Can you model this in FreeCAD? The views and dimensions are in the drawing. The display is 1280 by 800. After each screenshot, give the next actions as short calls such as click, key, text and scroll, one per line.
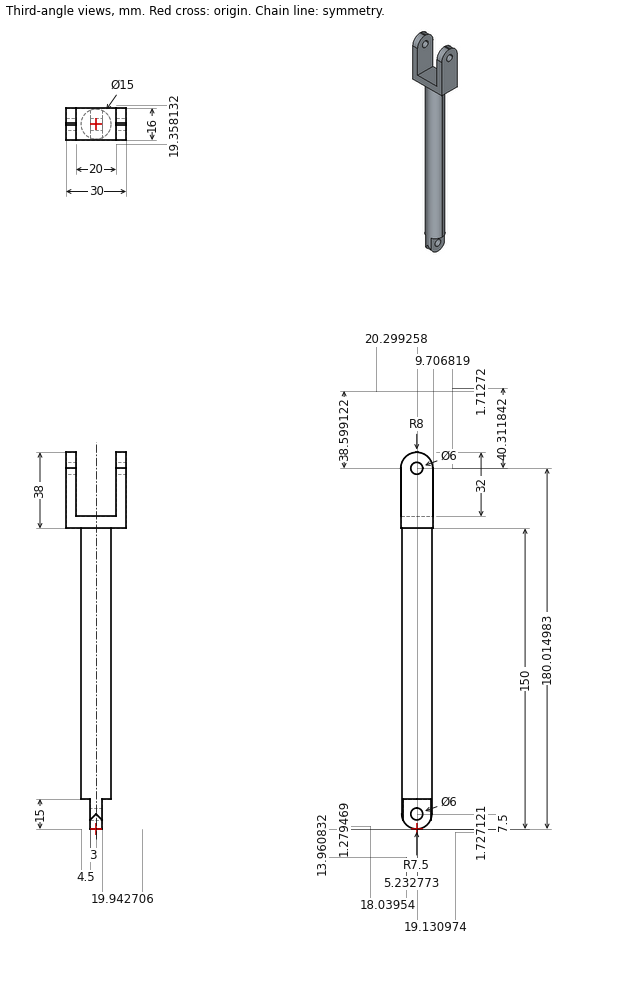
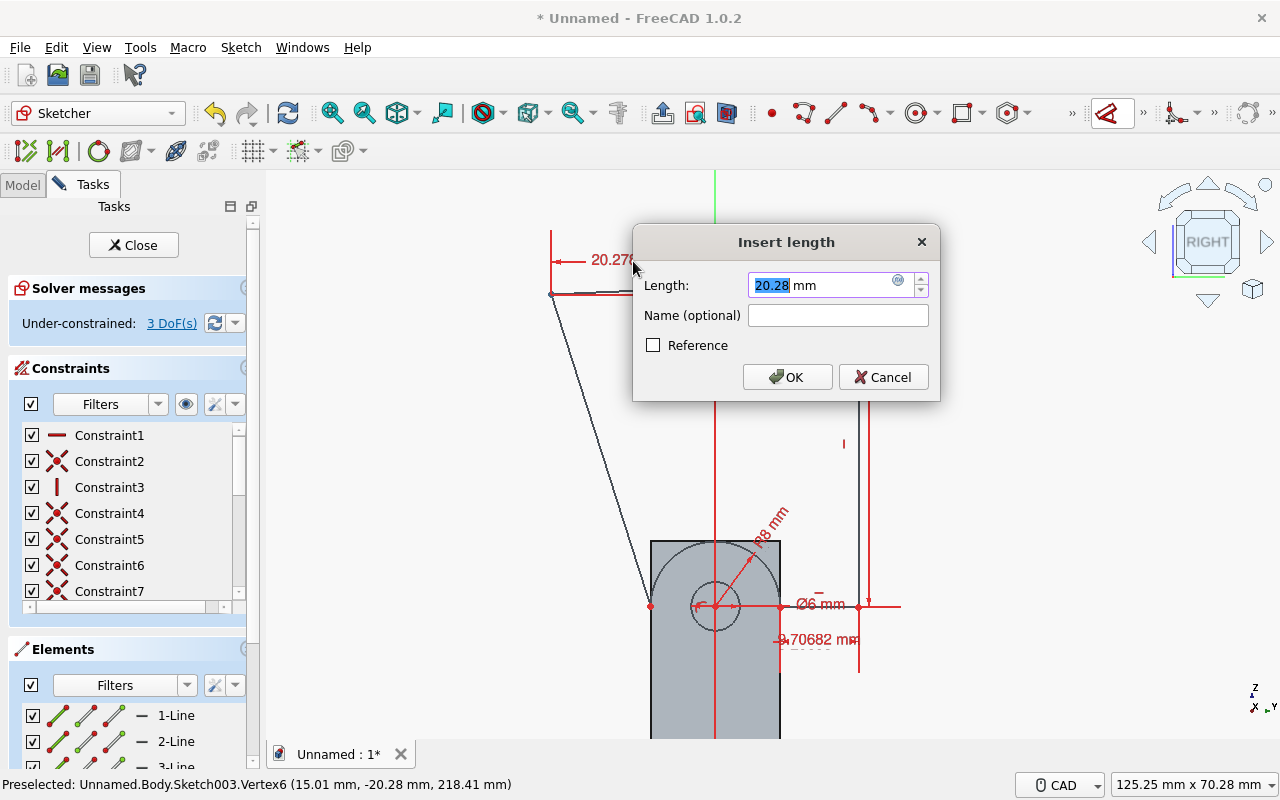
text(20.299258)
key(Return)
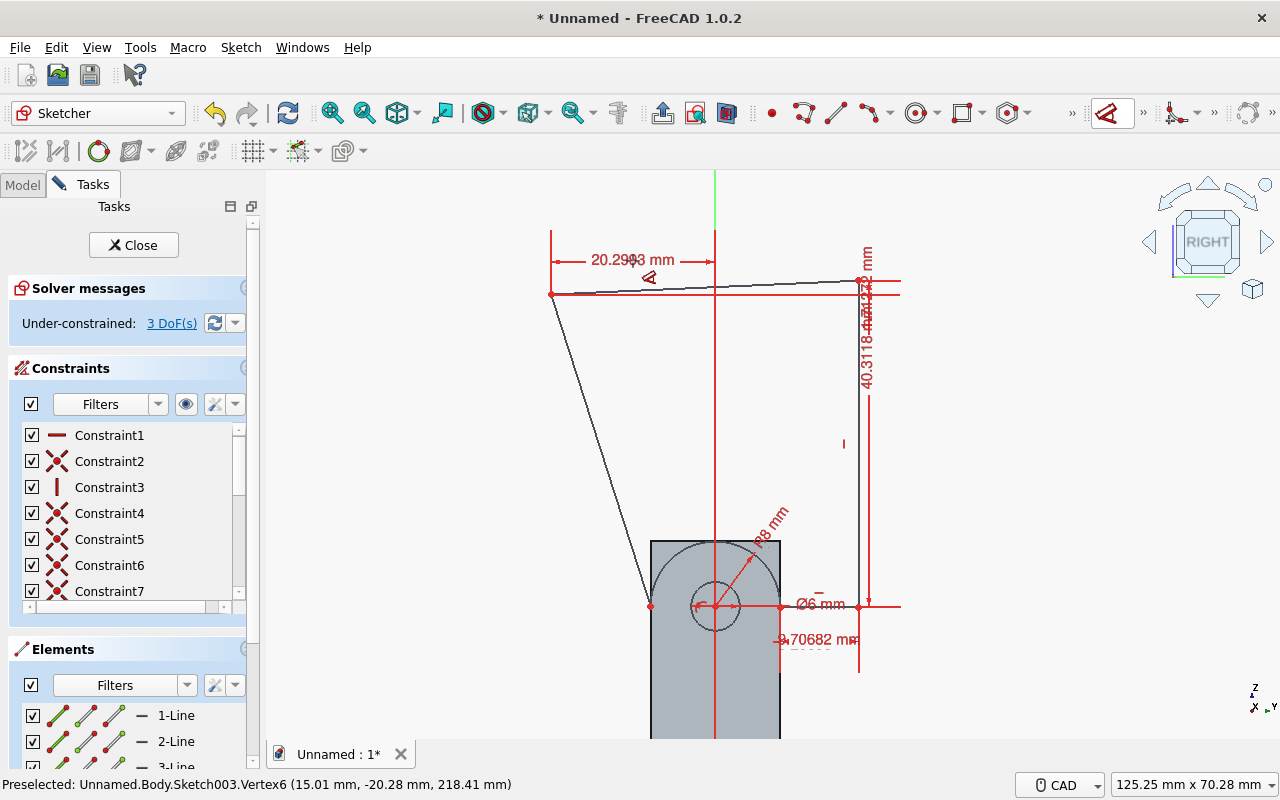
click(581, 388)
click(517, 450)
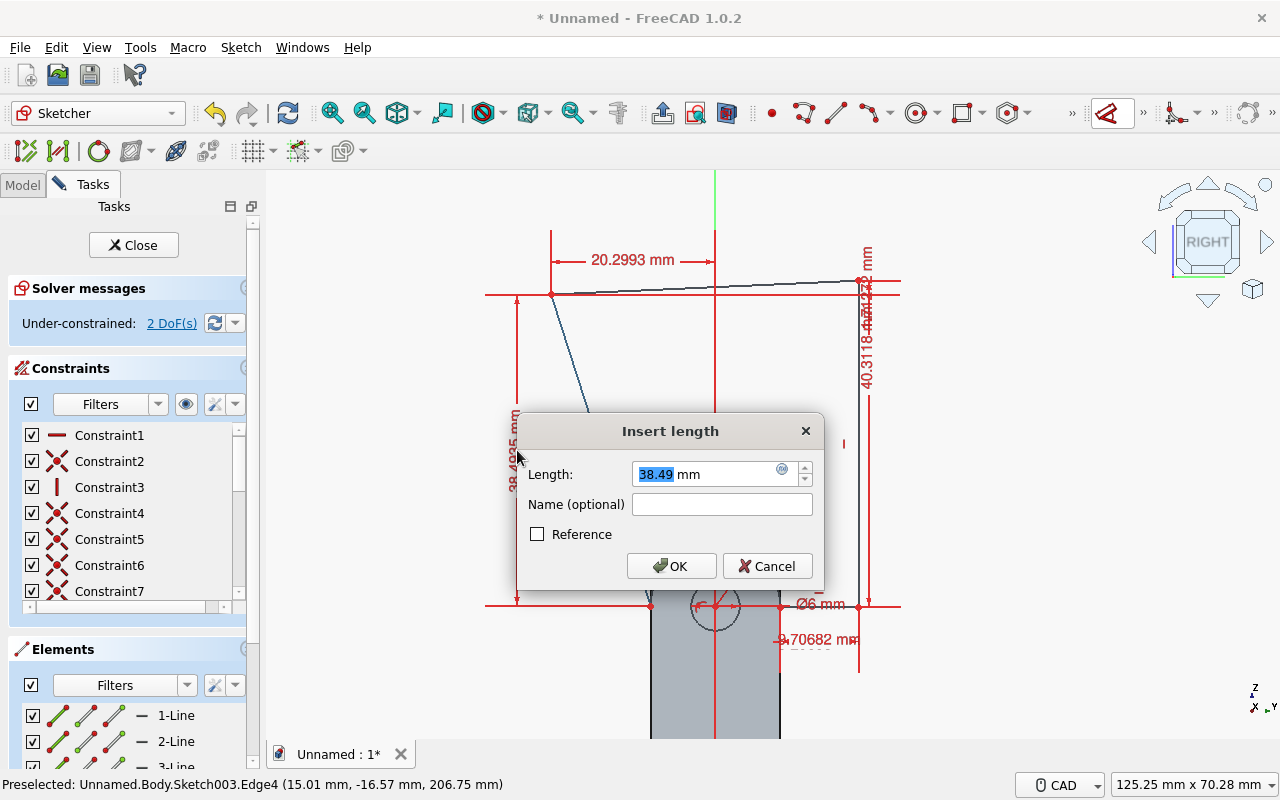
text(38.599122)
key(Return)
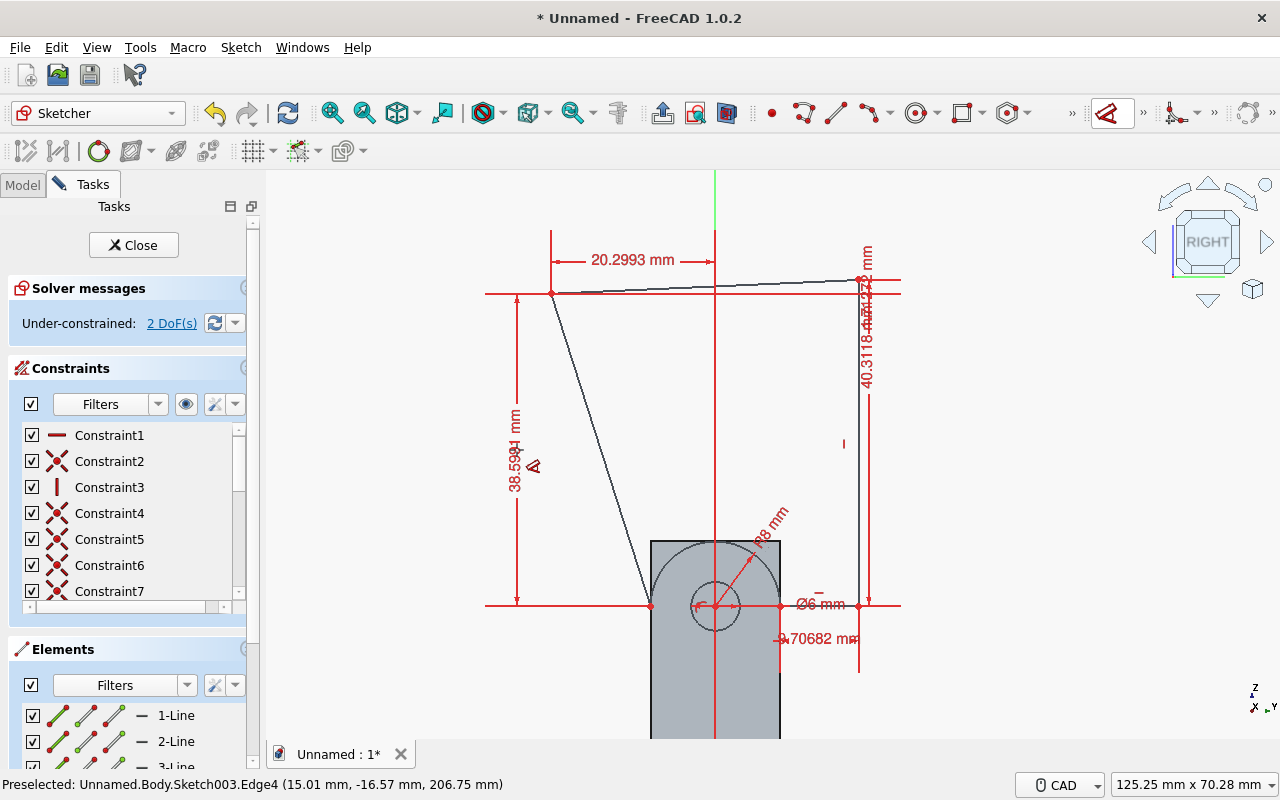
click(715, 606)
click(749, 659)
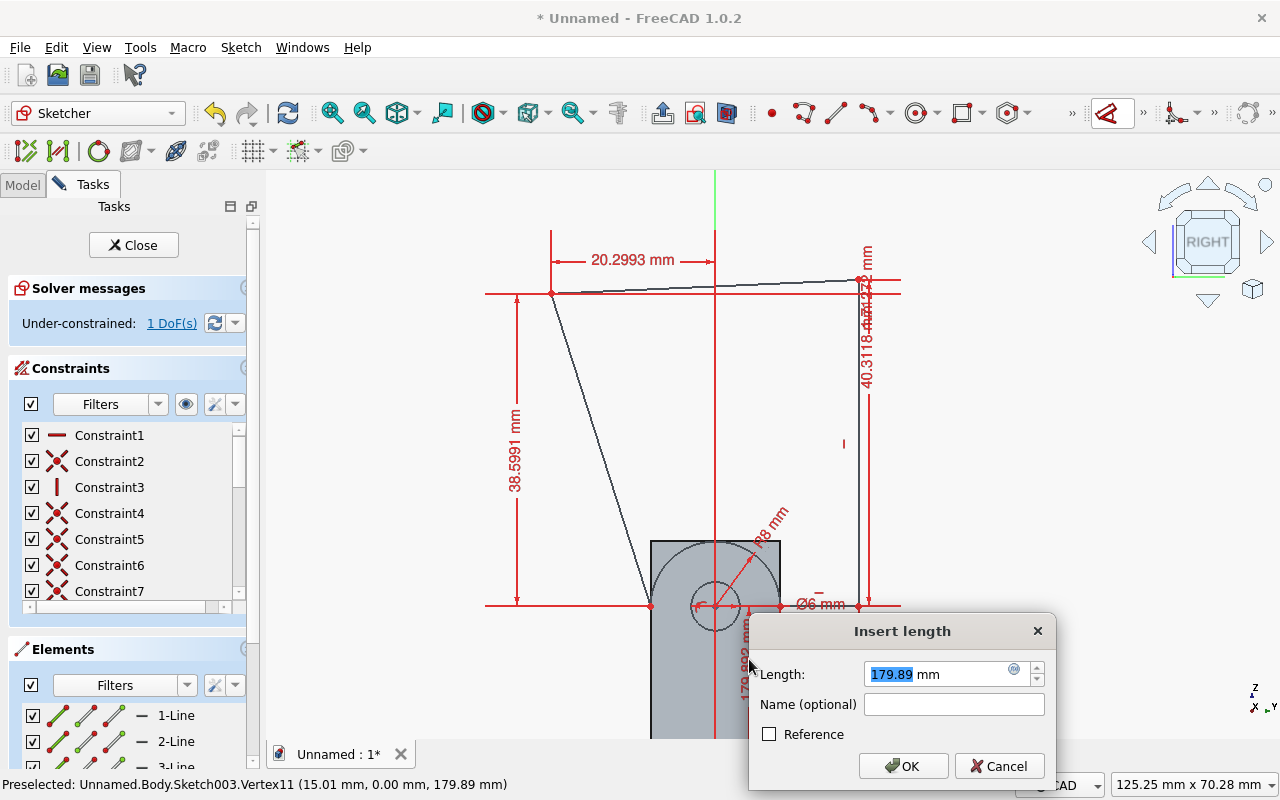
text(180.014983)
key(Return)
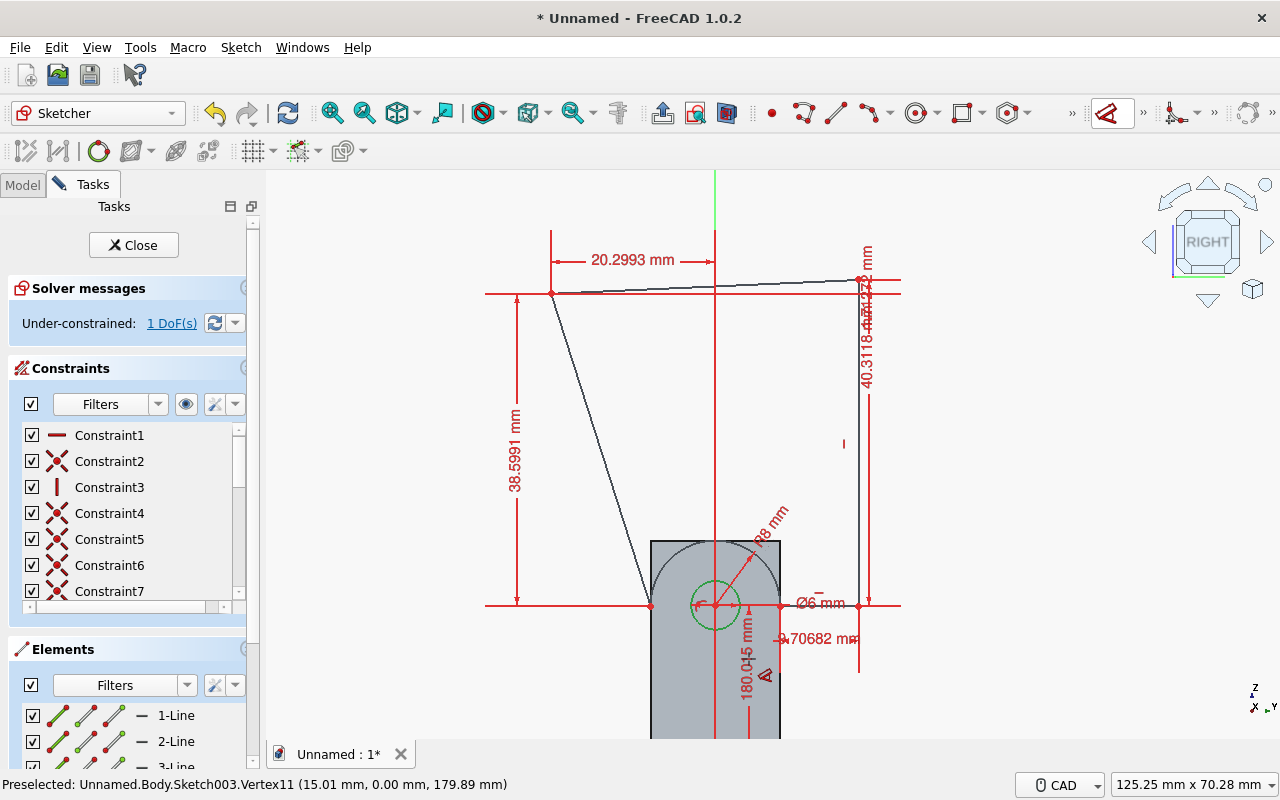
click(780, 606)
click(814, 683)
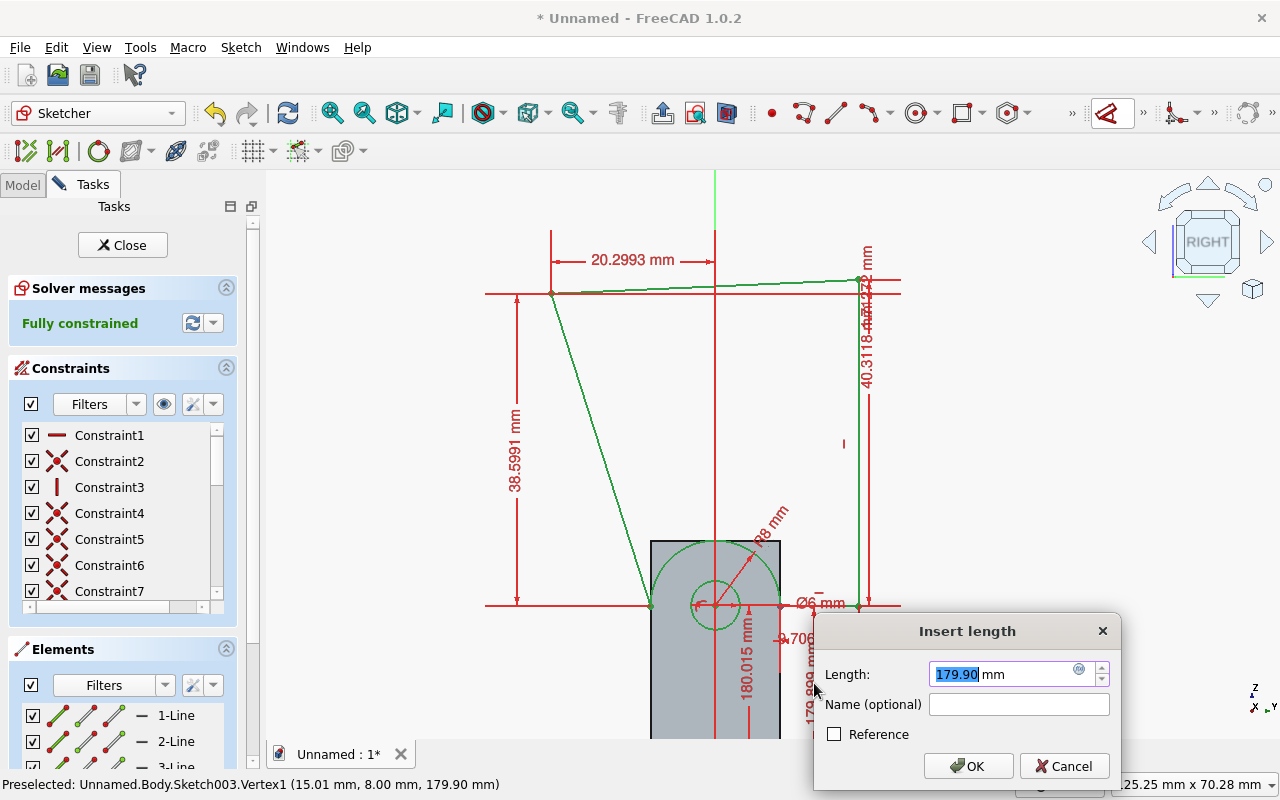
text(180.014983)
key(Return)
key(Escape)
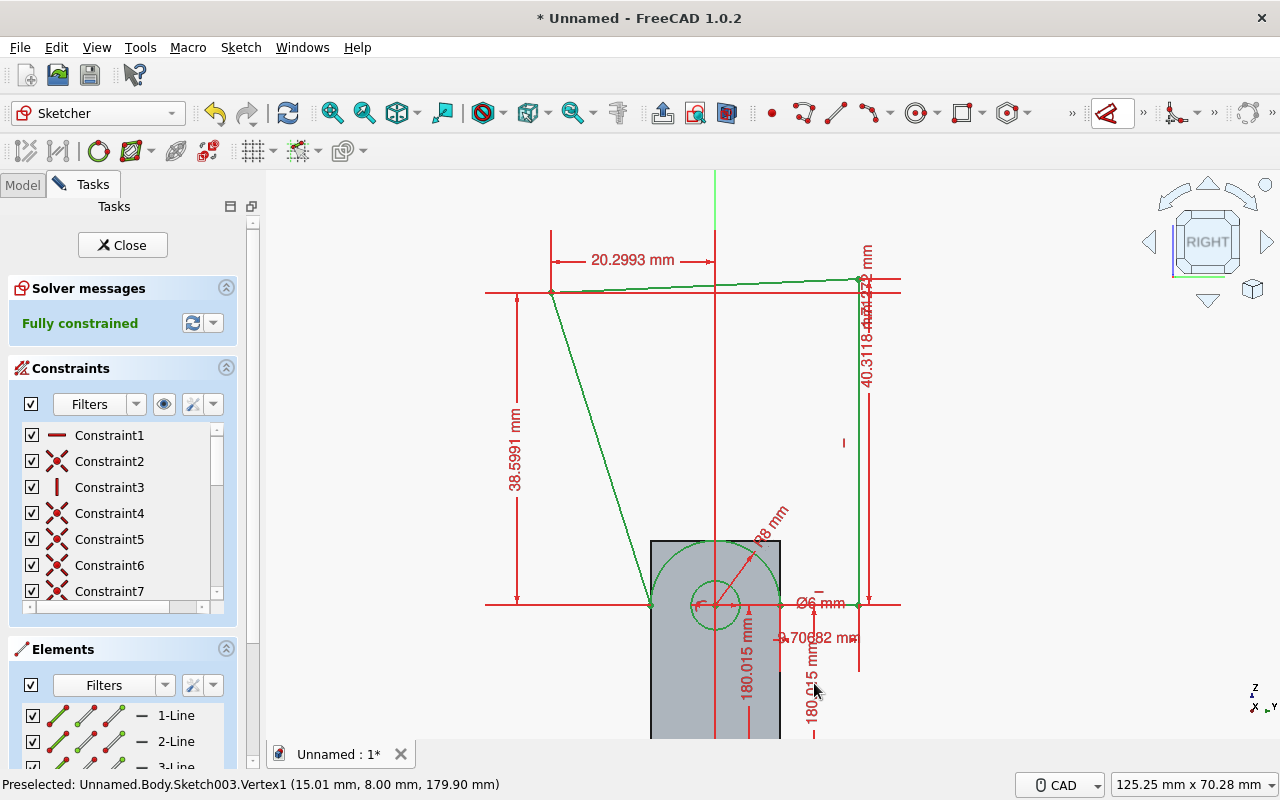
click(123, 245)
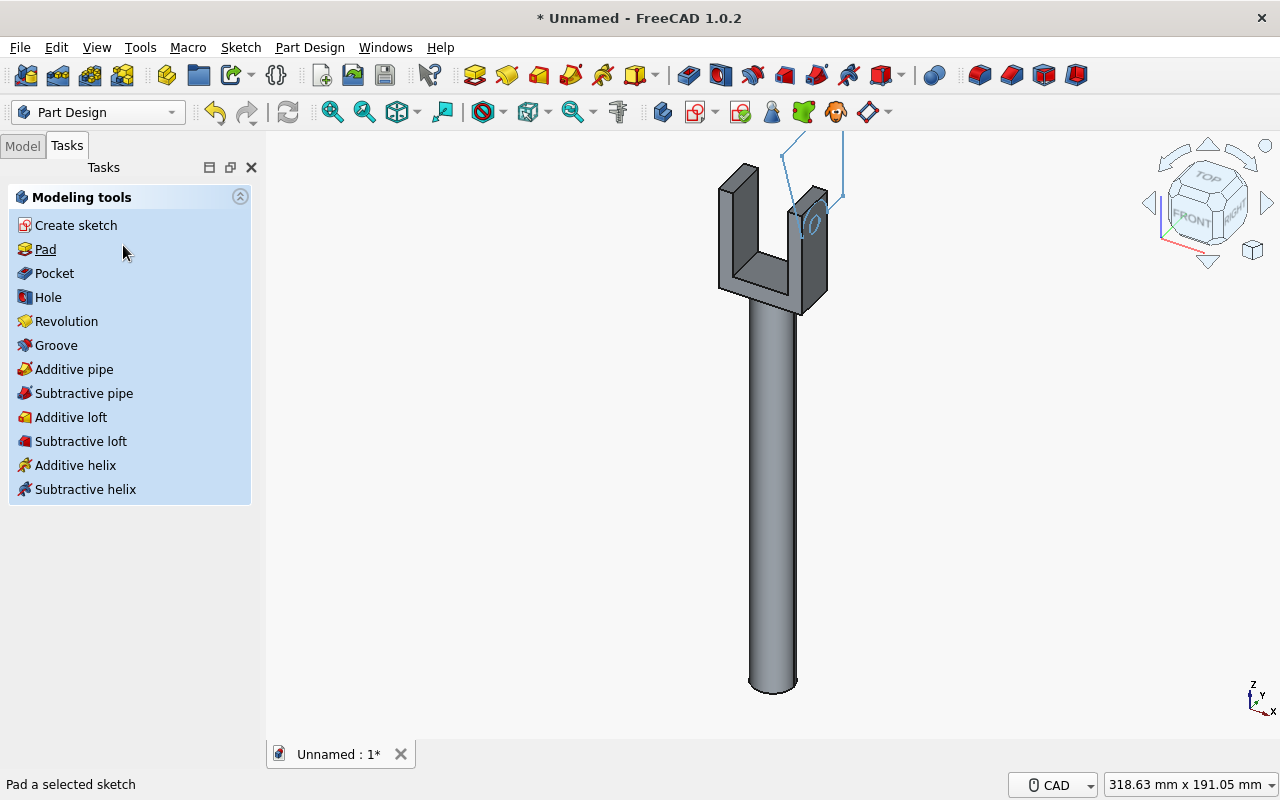
click(690, 76)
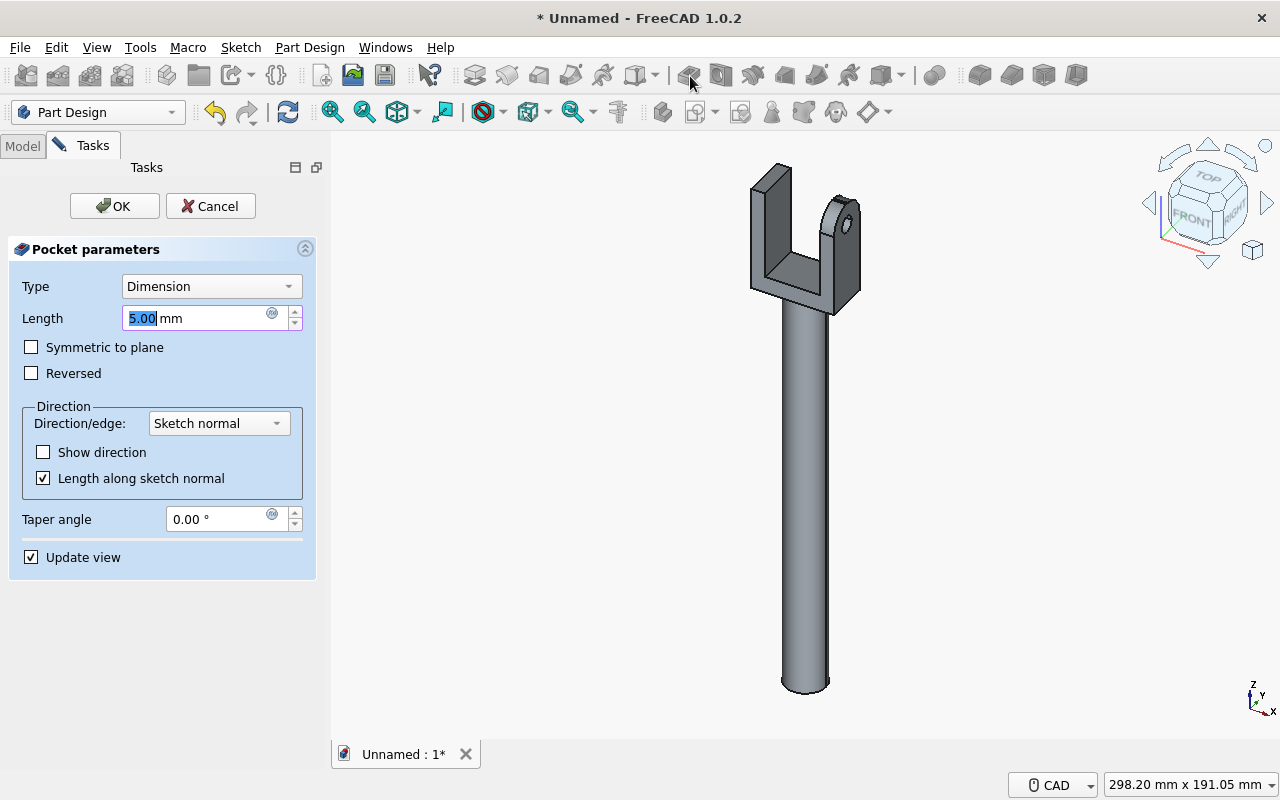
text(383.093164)
key(Tab)